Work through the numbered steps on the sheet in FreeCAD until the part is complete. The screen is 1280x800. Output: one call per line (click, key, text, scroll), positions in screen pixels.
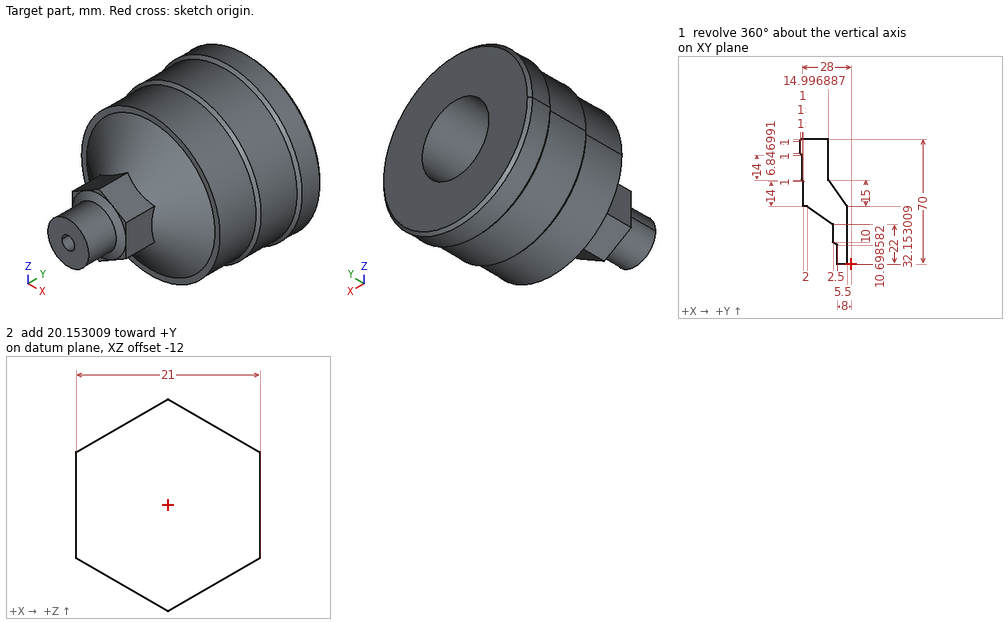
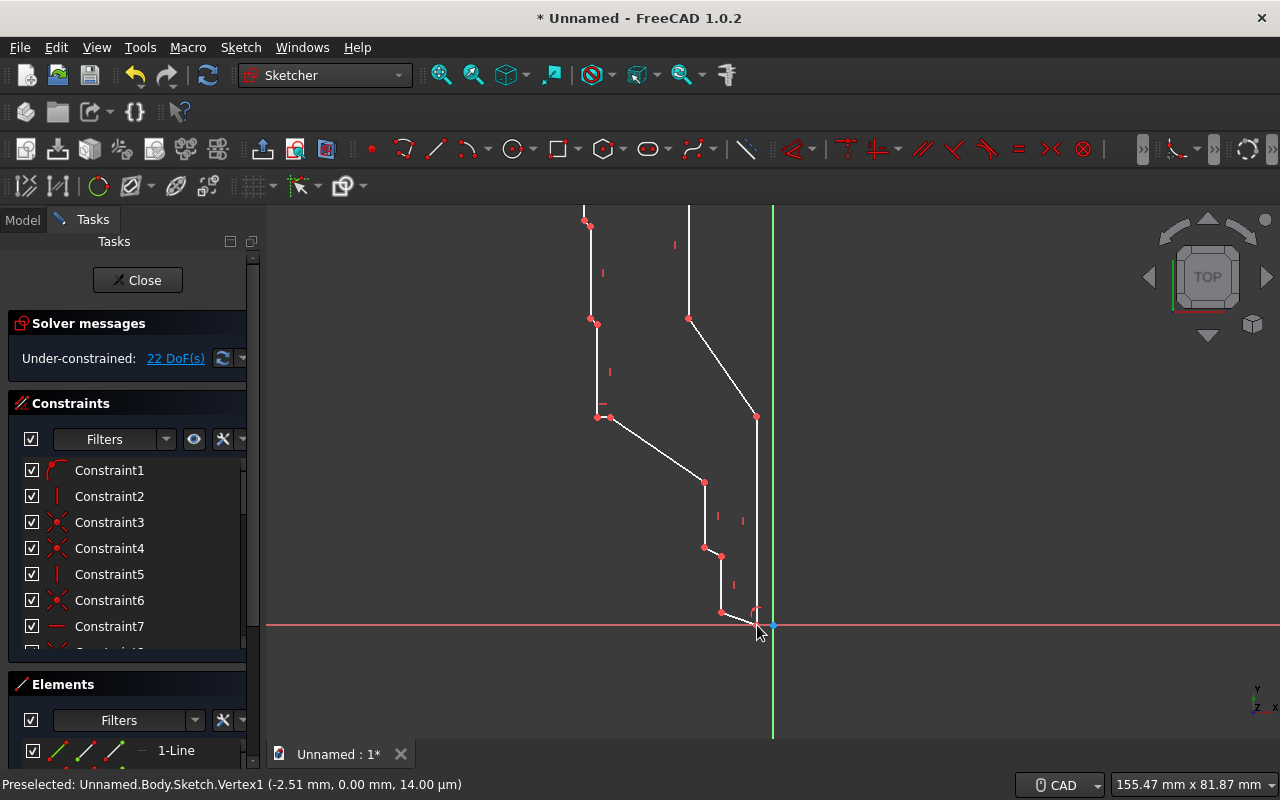
scroll(746, 621, up, 2)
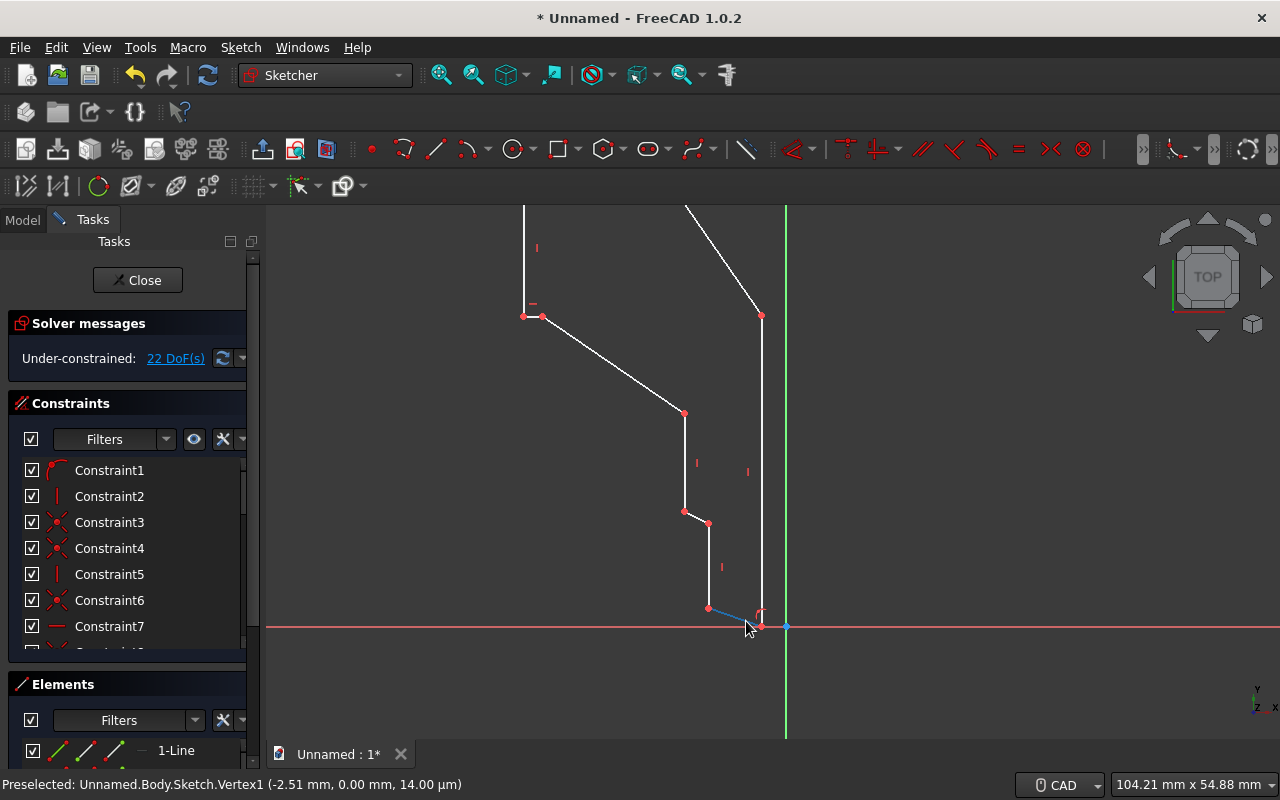
click(746, 621)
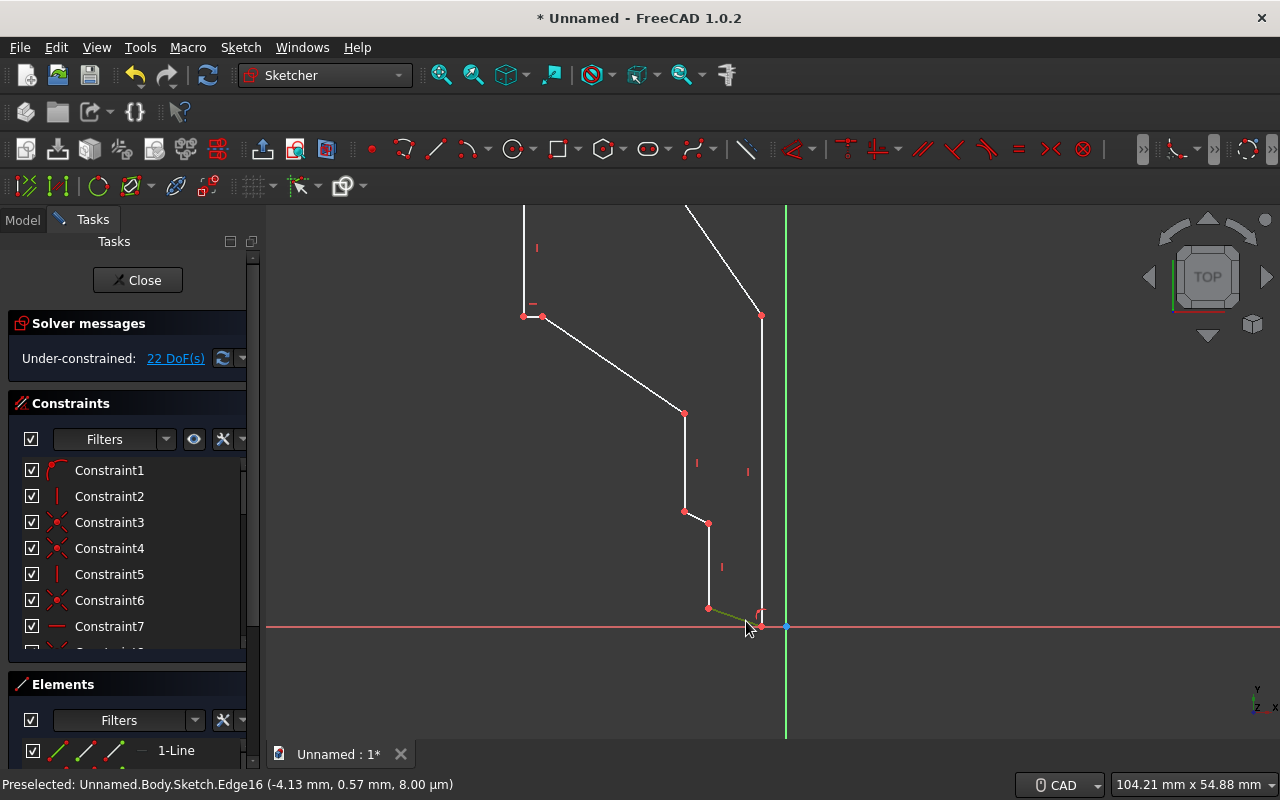
click(900, 150)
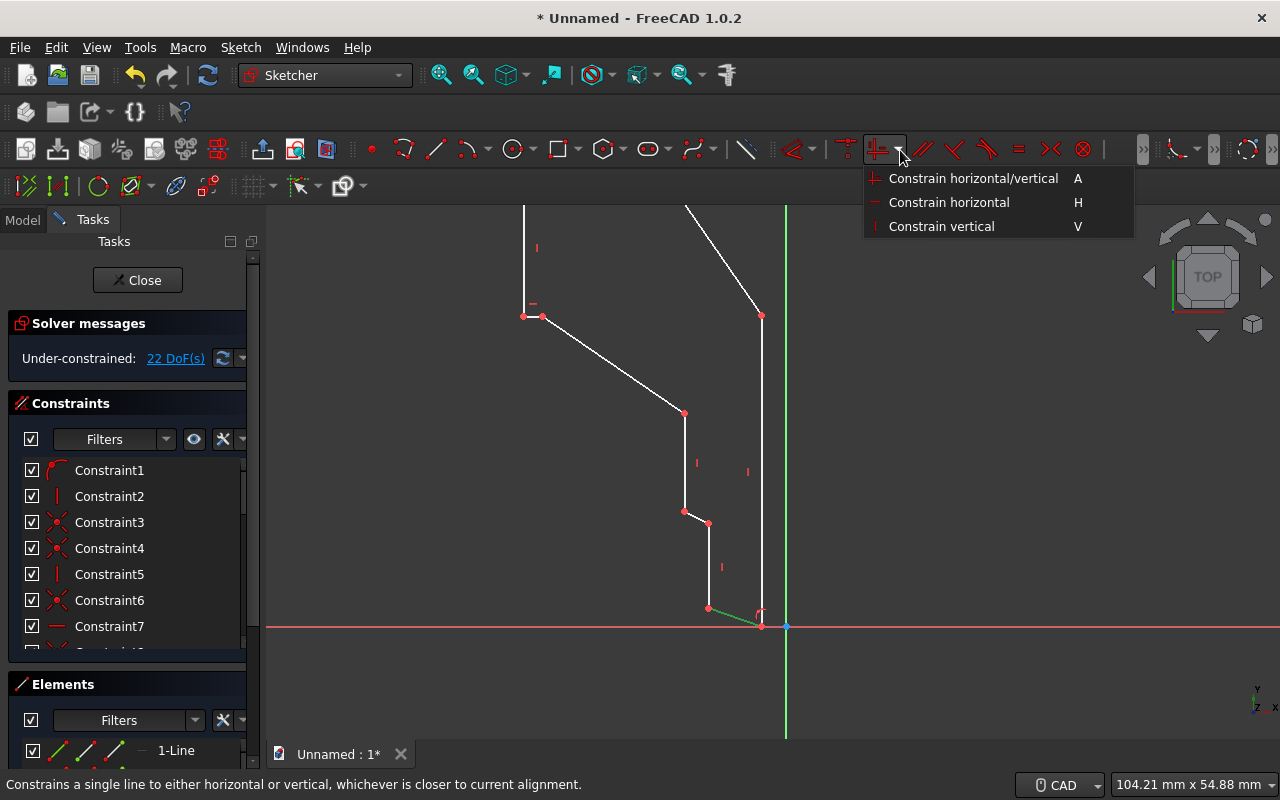
click(999, 202)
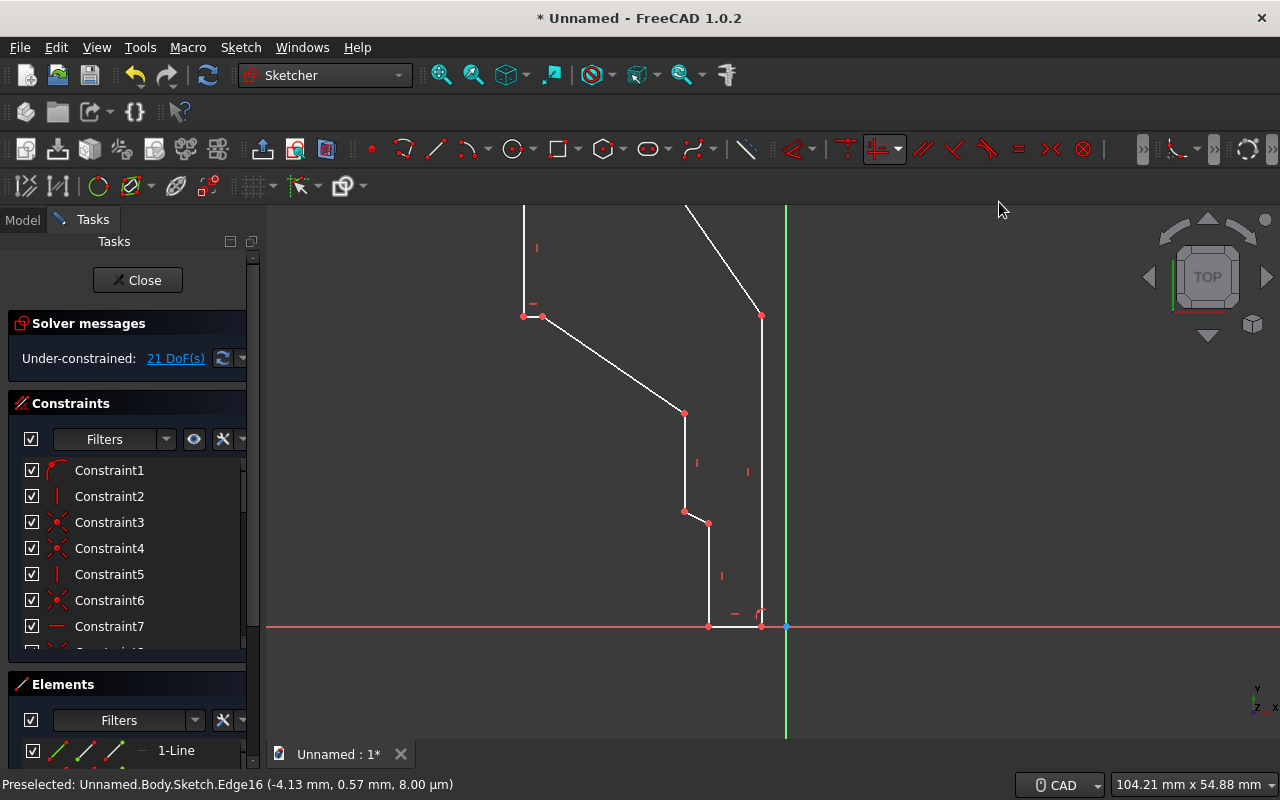
scroll(533, 317, up, 4)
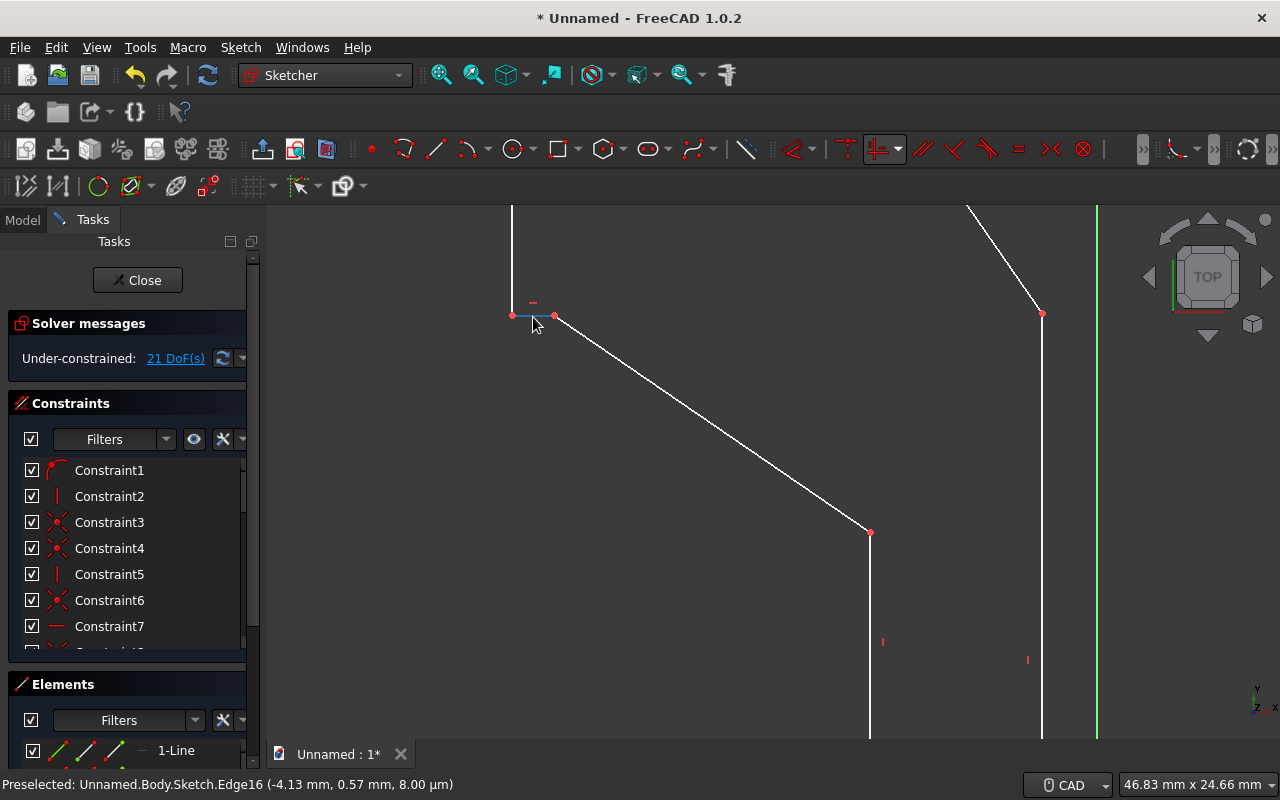
click(533, 316)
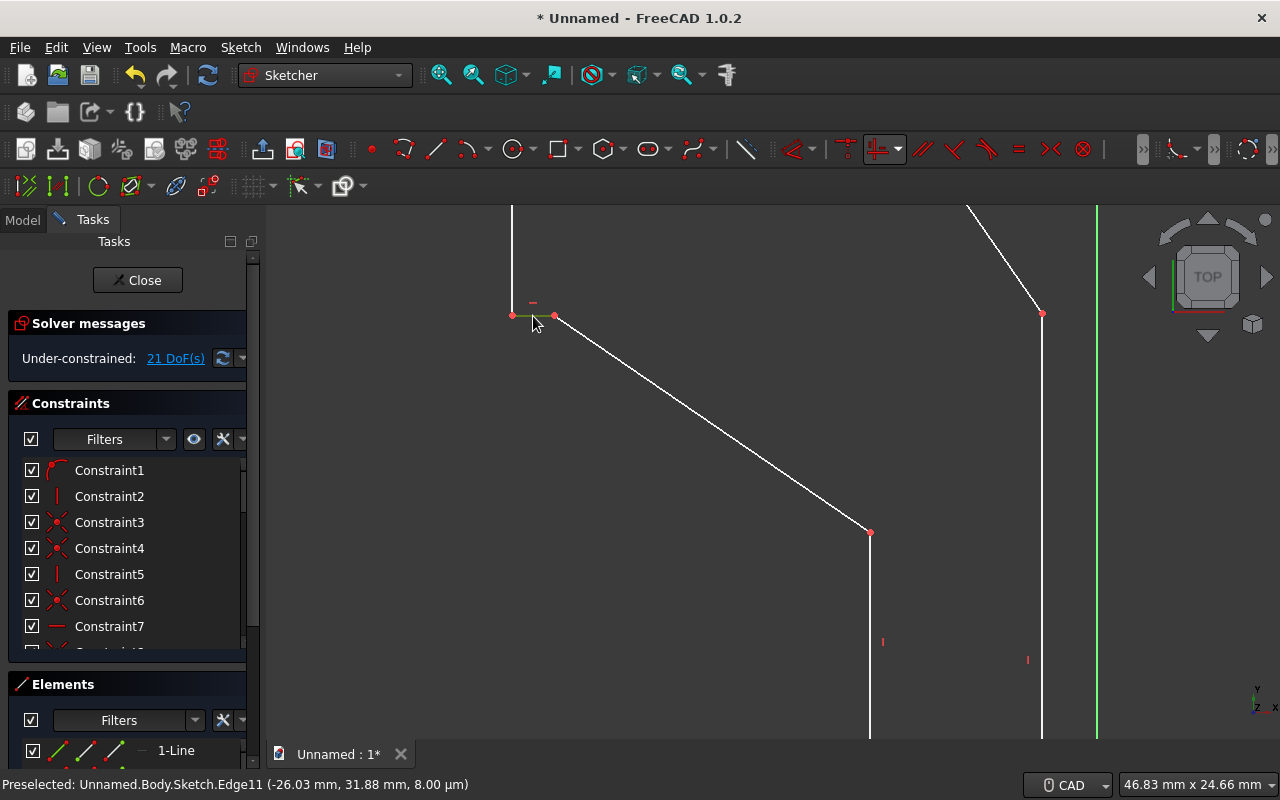
click(814, 150)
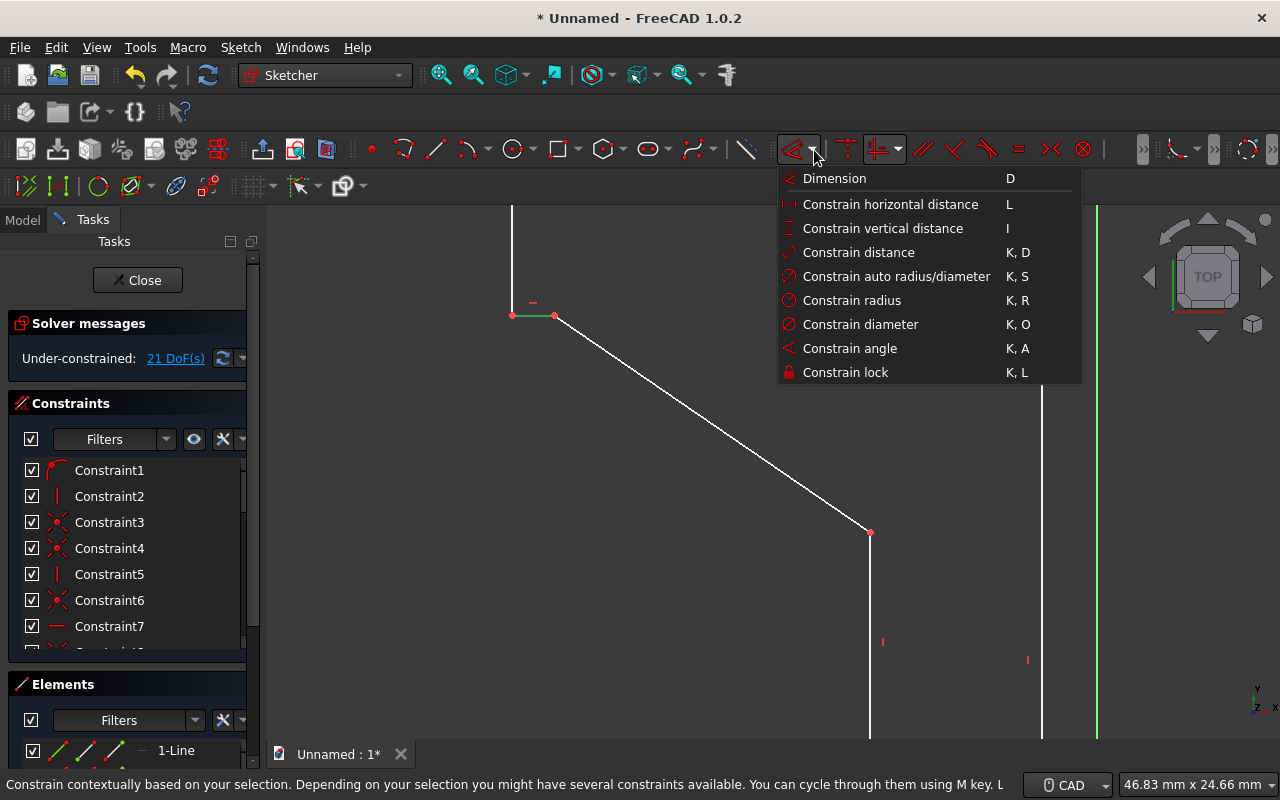
click(930, 204)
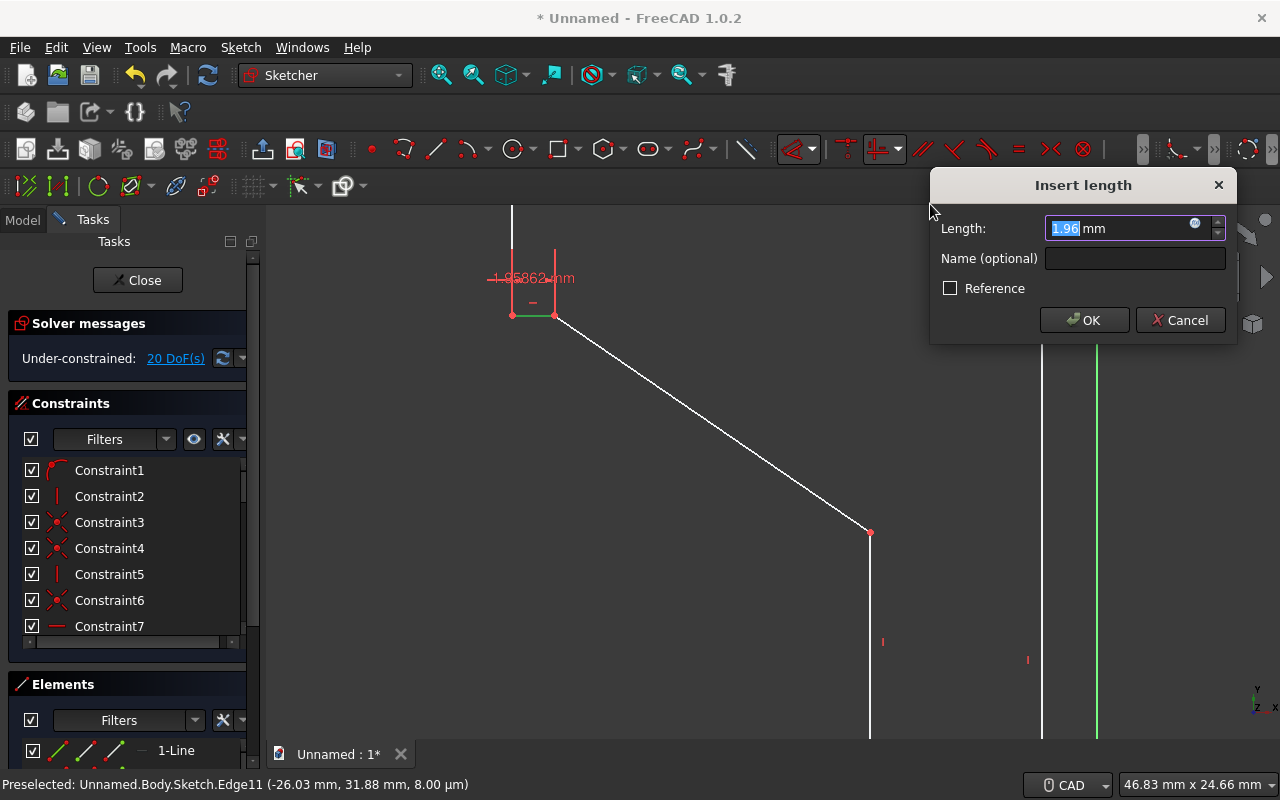
text(2)
key(Return)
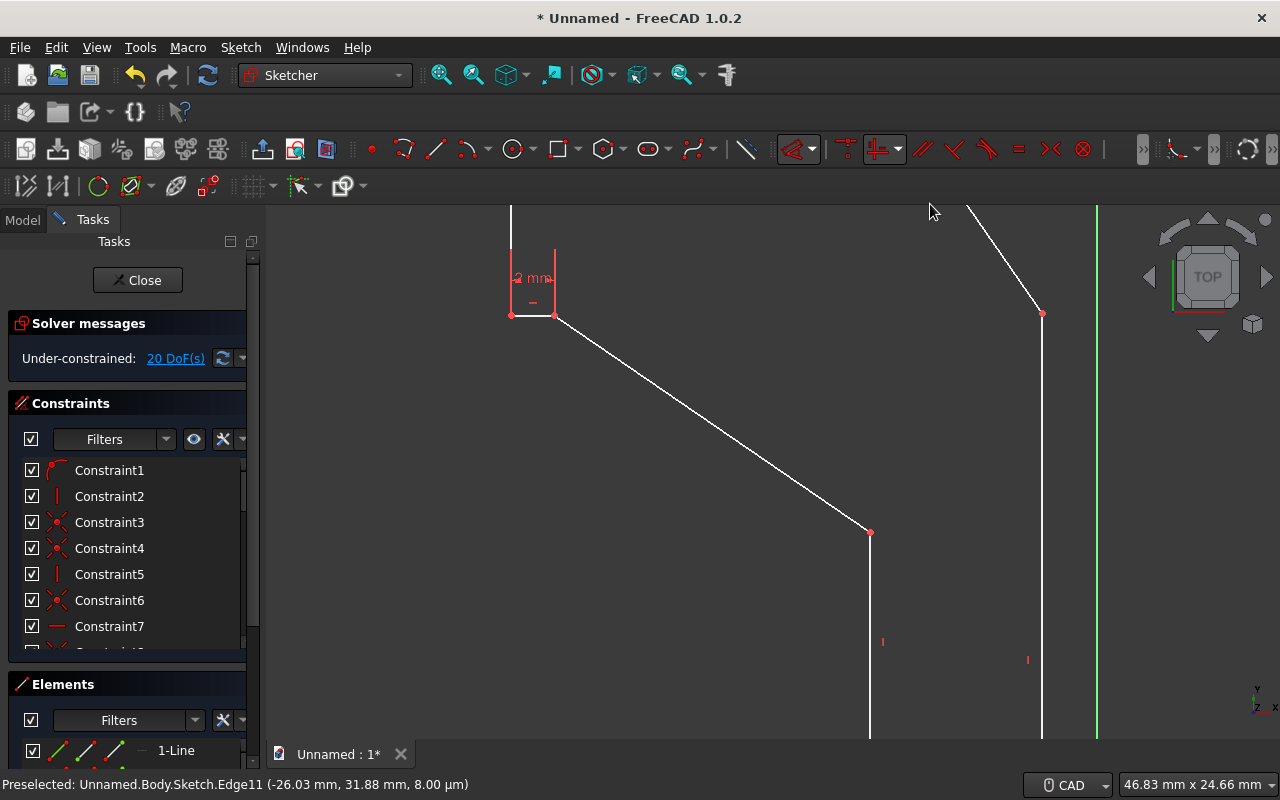
scroll(685, 529, down, 8)